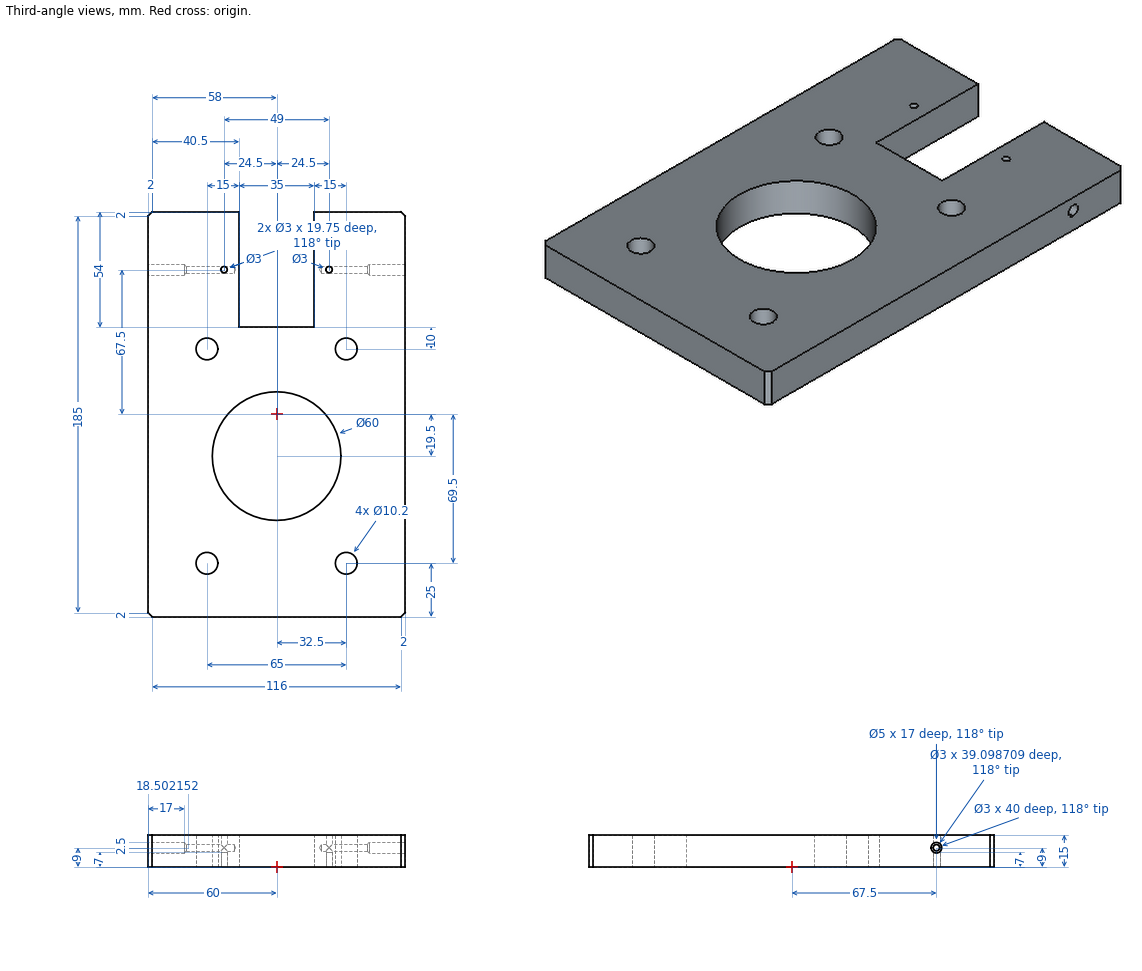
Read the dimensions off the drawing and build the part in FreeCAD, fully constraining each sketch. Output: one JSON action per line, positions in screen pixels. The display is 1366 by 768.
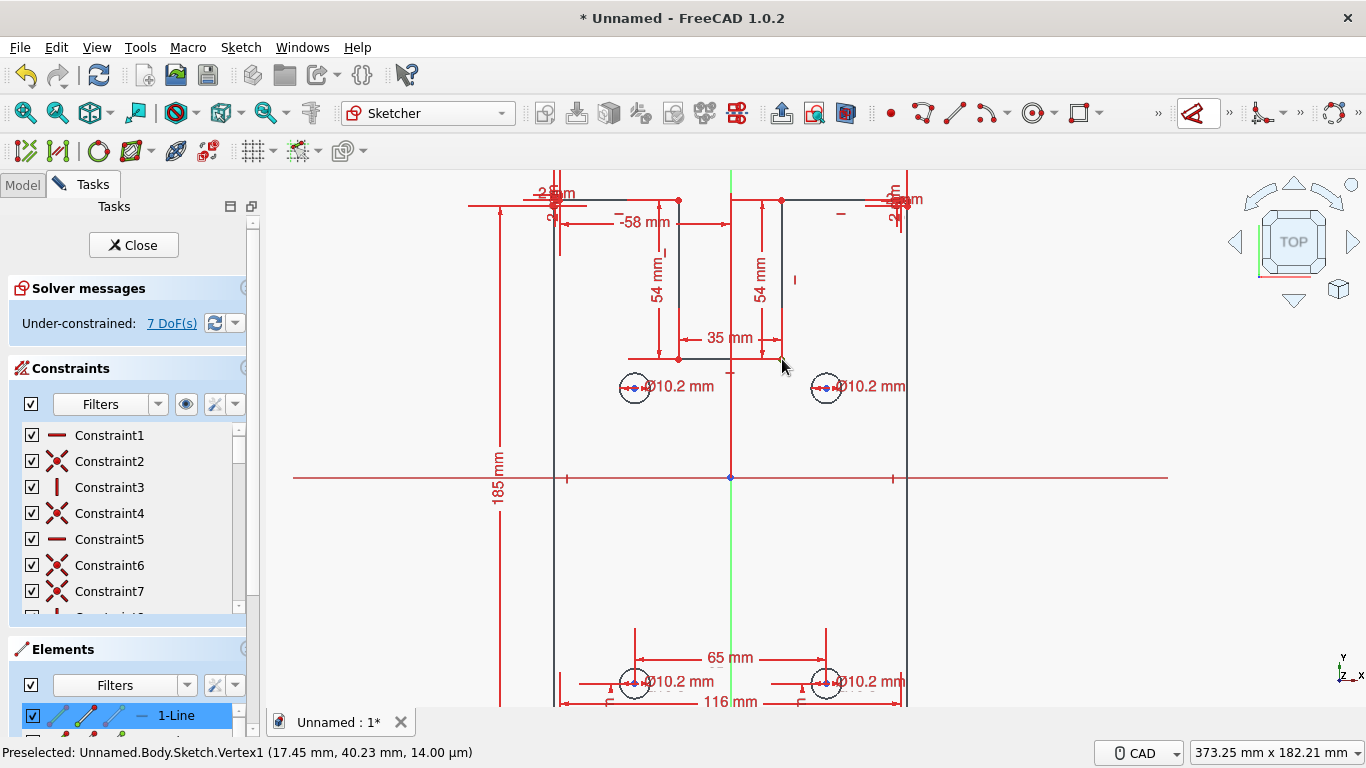
{"action": "left_click", "coordinate": [826, 388]}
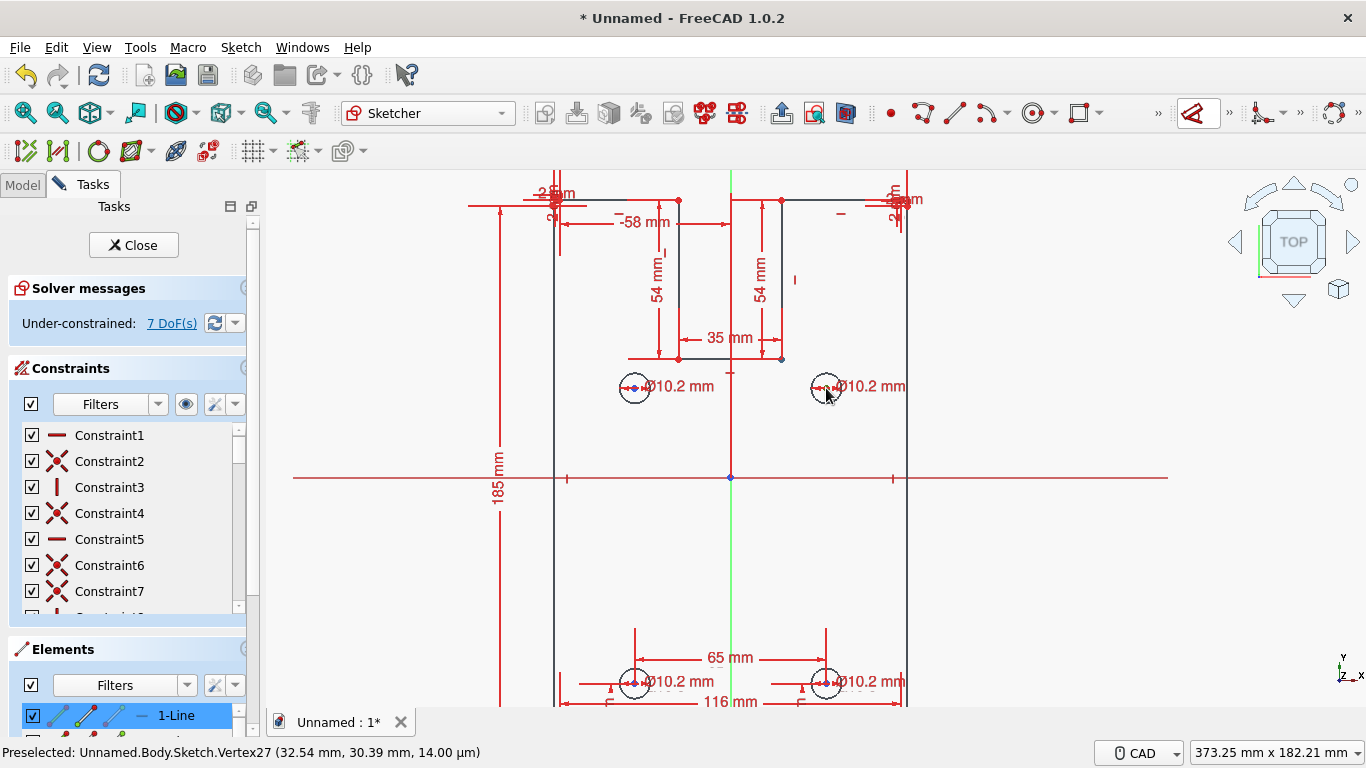
{"action": "key", "text": "l"}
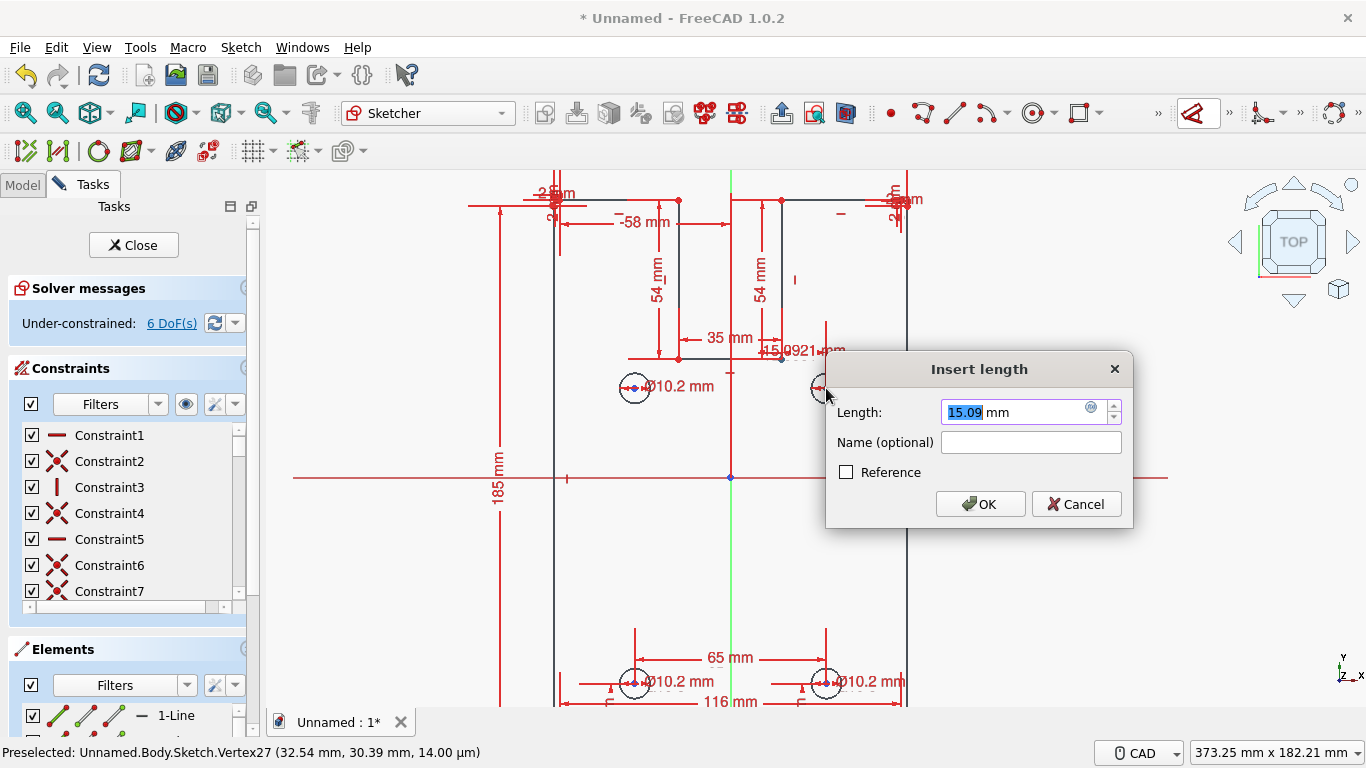
{"action": "type", "text": "15"}
{"action": "key", "text": "Return"}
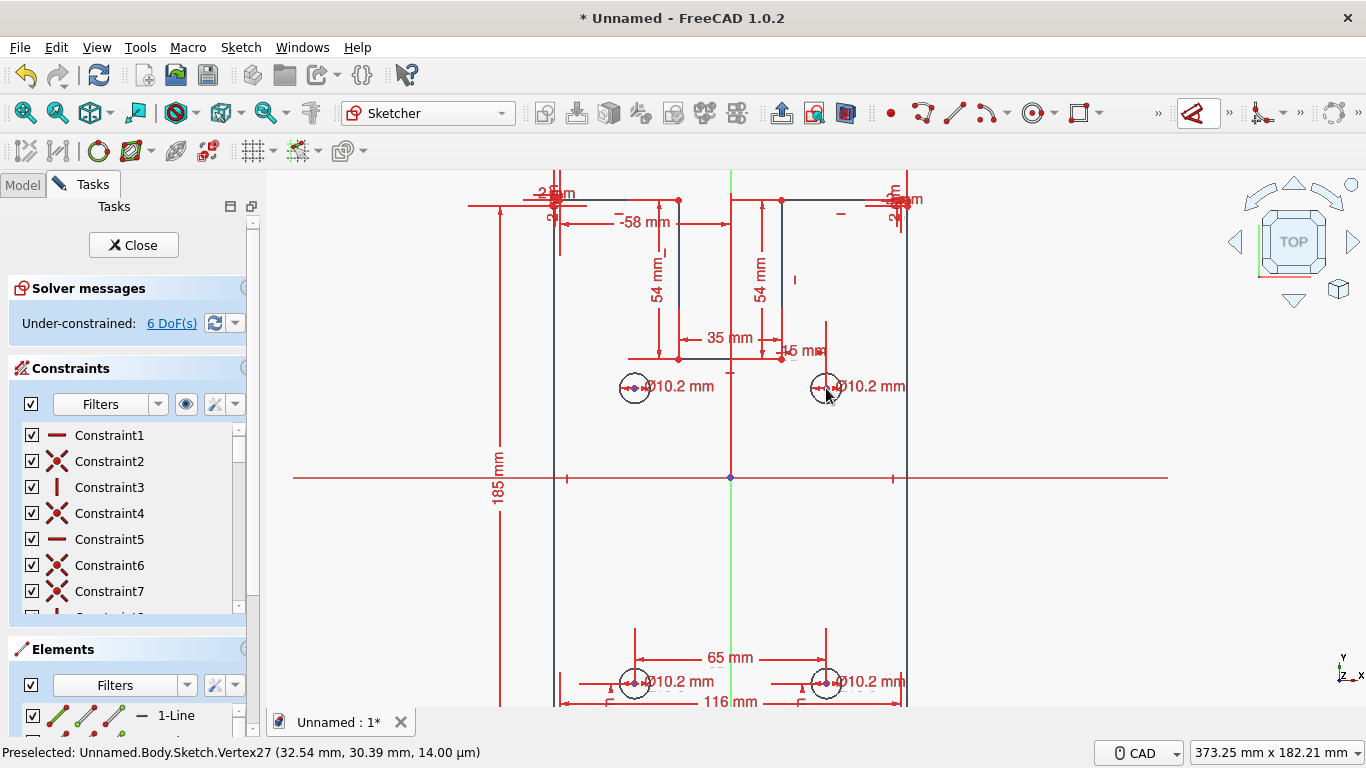
{"action": "scroll", "coordinate": [782, 359], "scroll_direction": "up", "scroll_amount": 2}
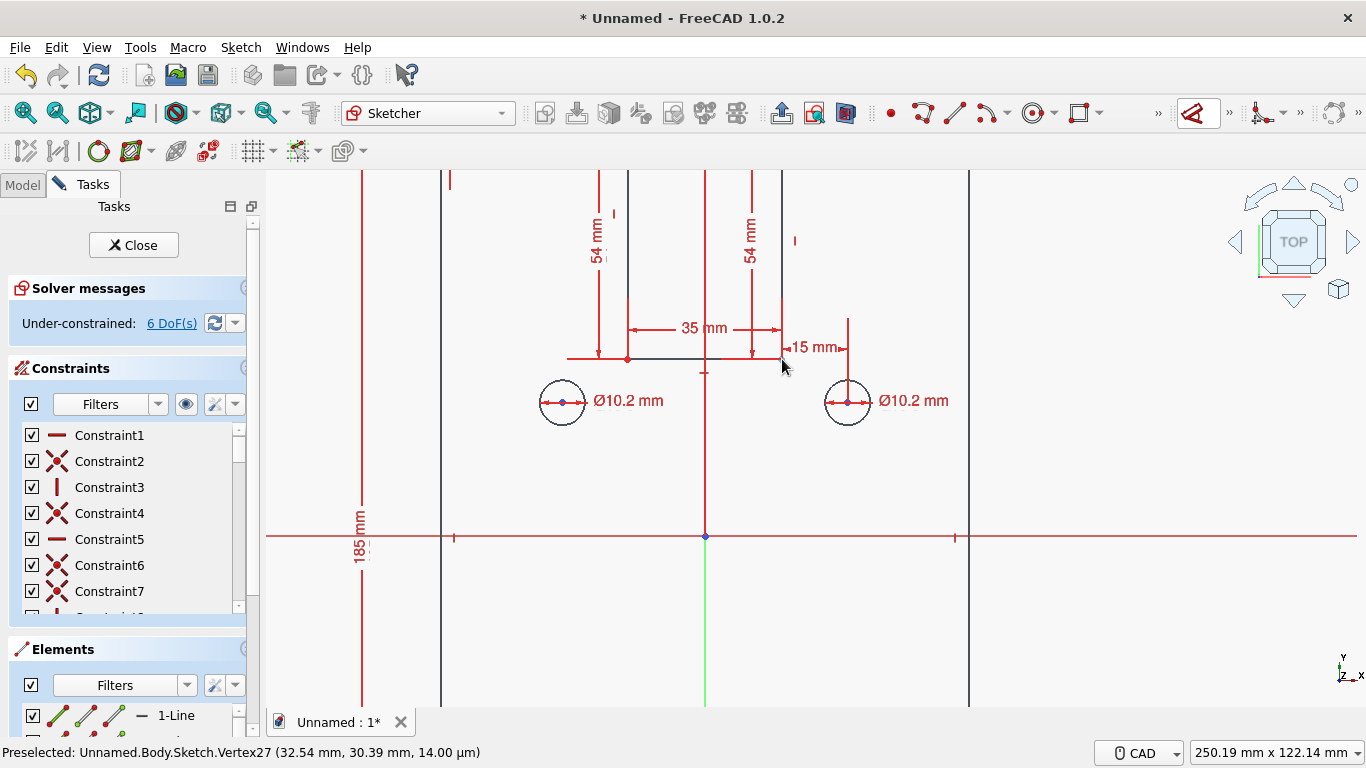
{"action": "left_click", "coordinate": [782, 359]}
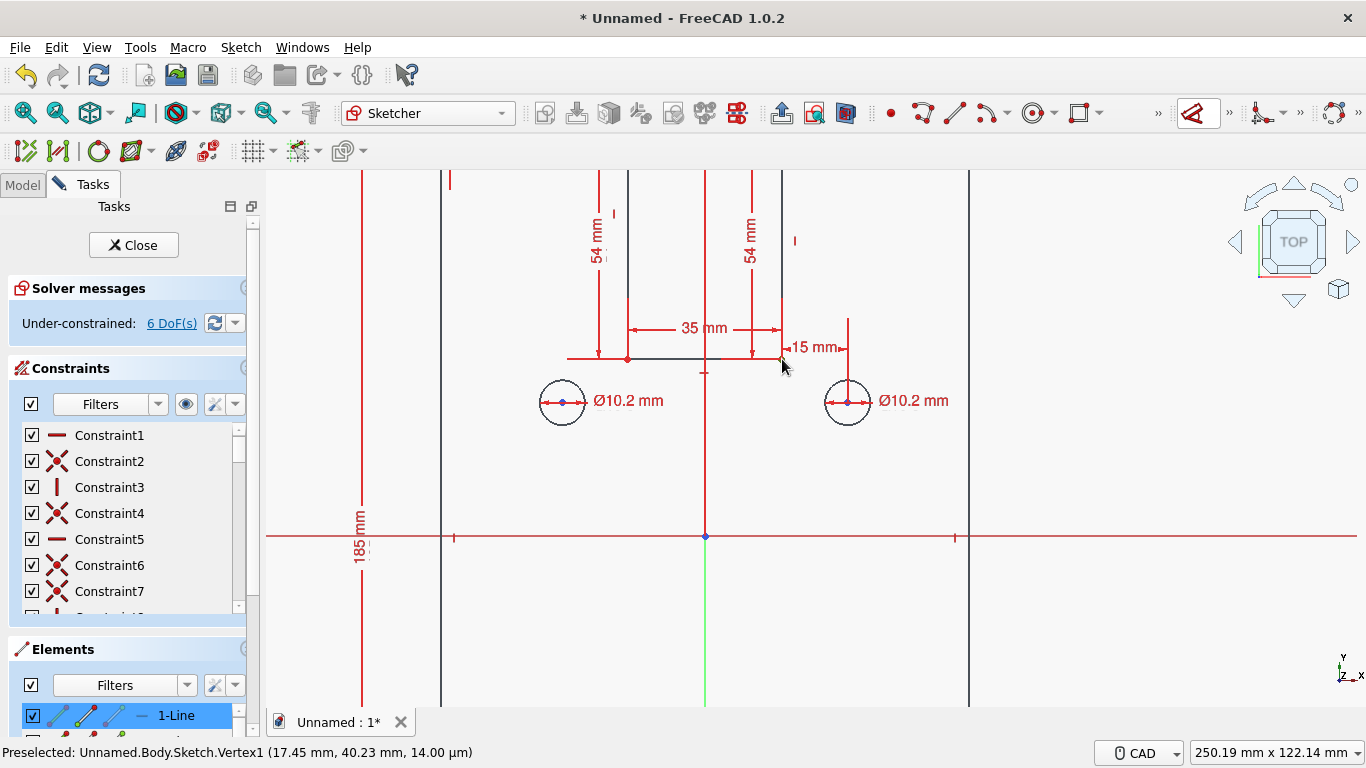
{"action": "left_click", "coordinate": [848, 403]}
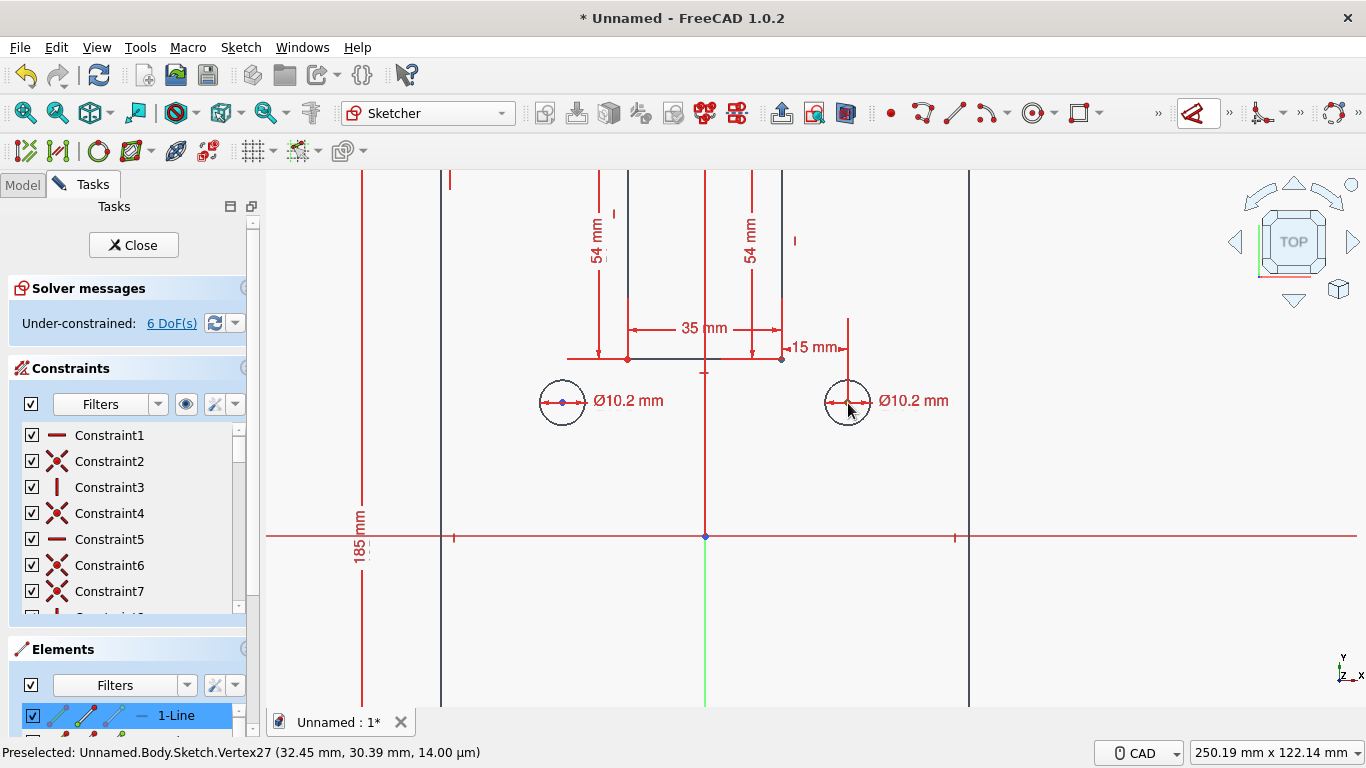
{"action": "left_click", "coordinate": [1214, 114]}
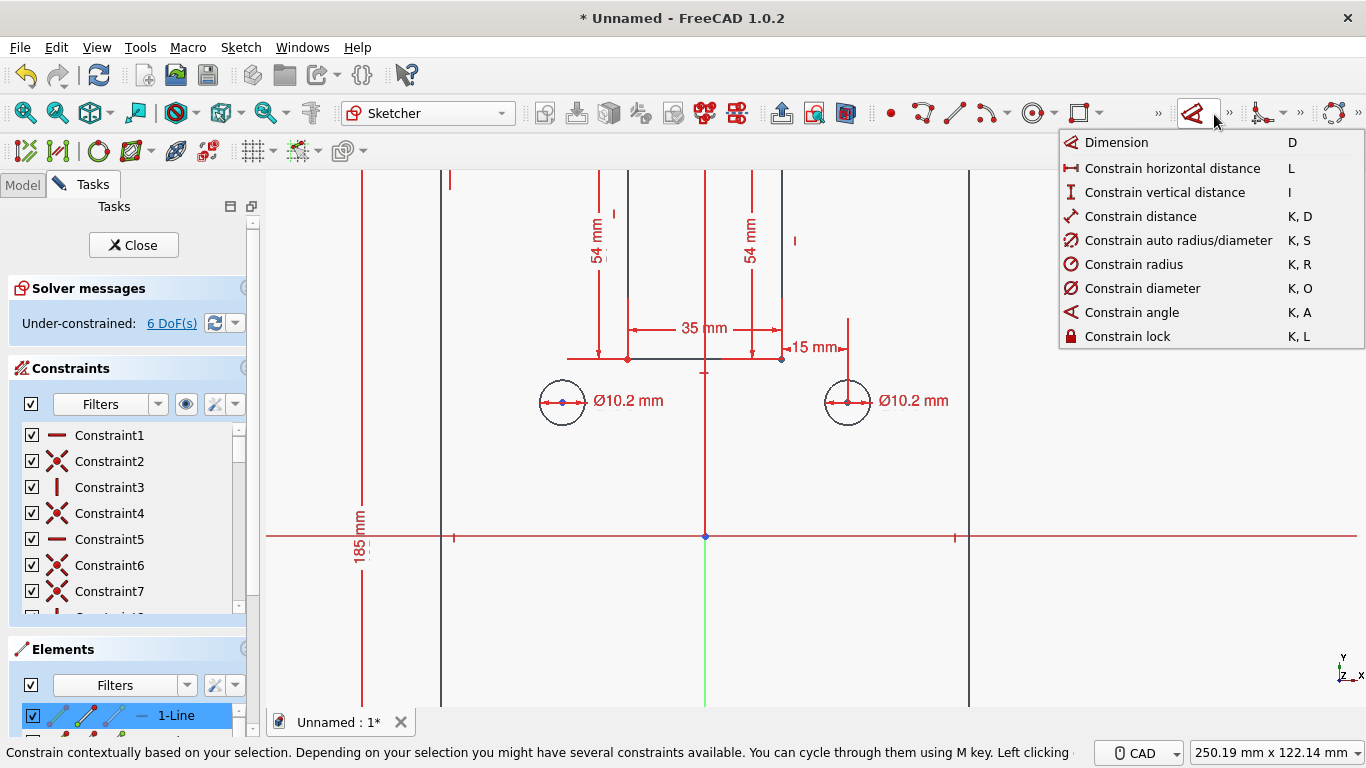
{"action": "left_click", "coordinate": [1212, 192]}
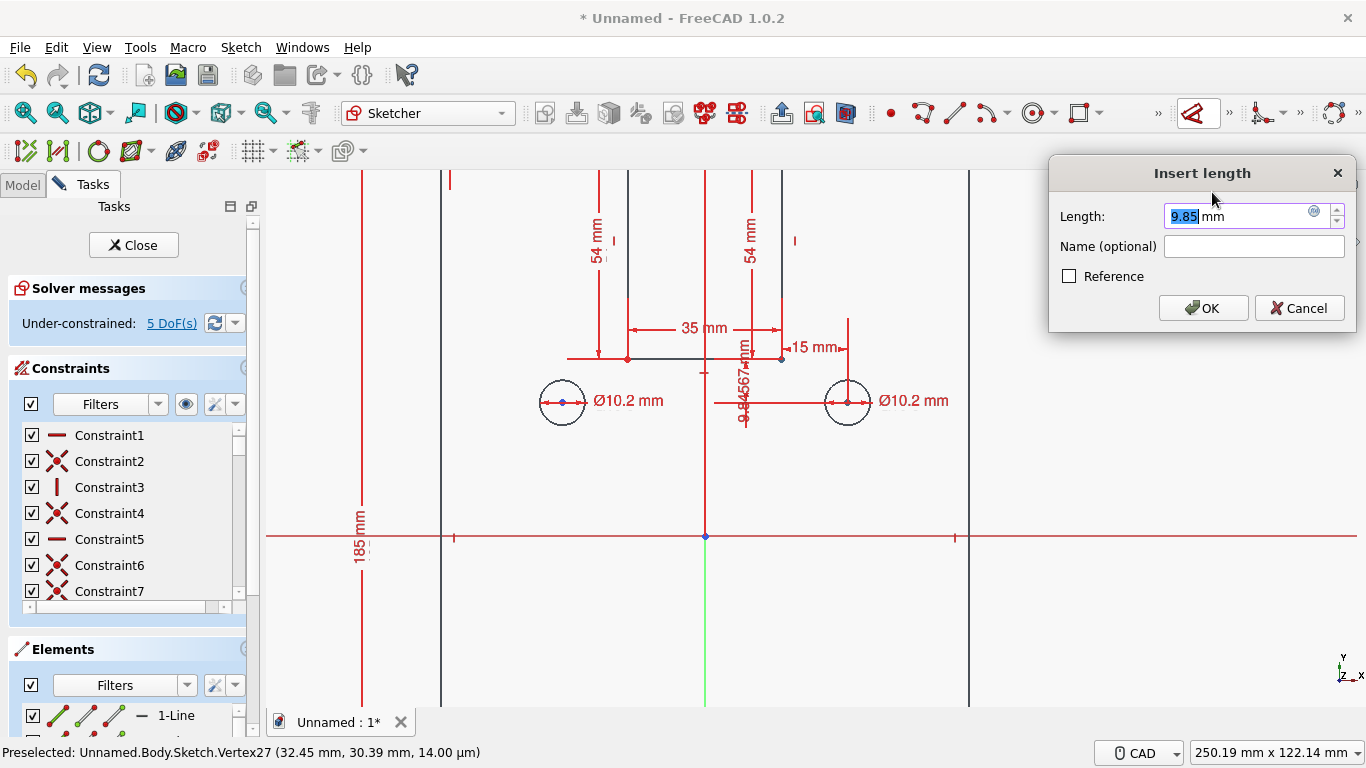
{"action": "type", "text": "10"}
{"action": "key", "text": "Return"}